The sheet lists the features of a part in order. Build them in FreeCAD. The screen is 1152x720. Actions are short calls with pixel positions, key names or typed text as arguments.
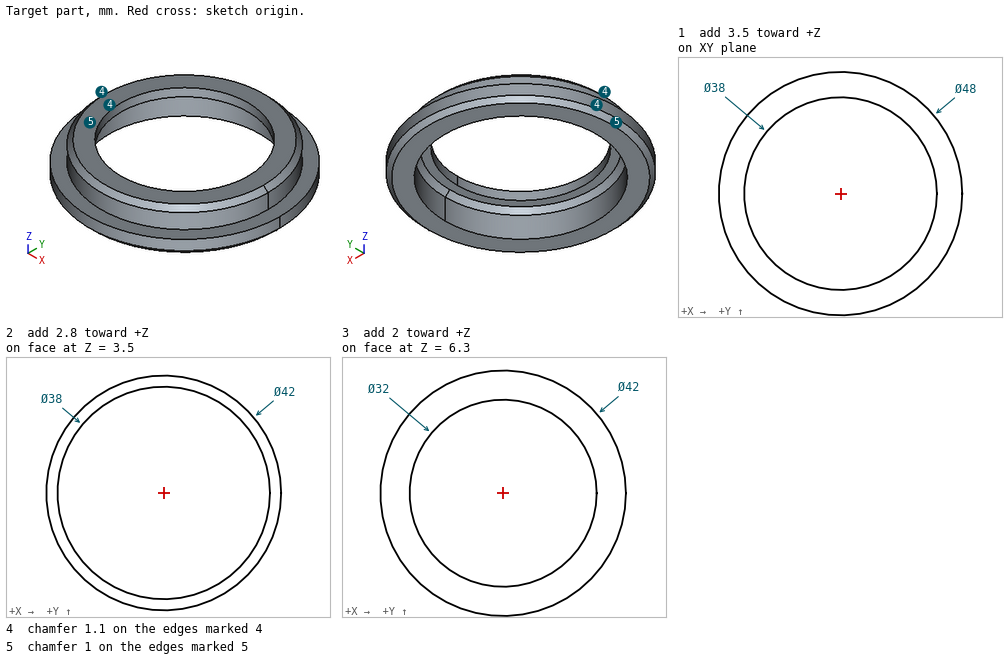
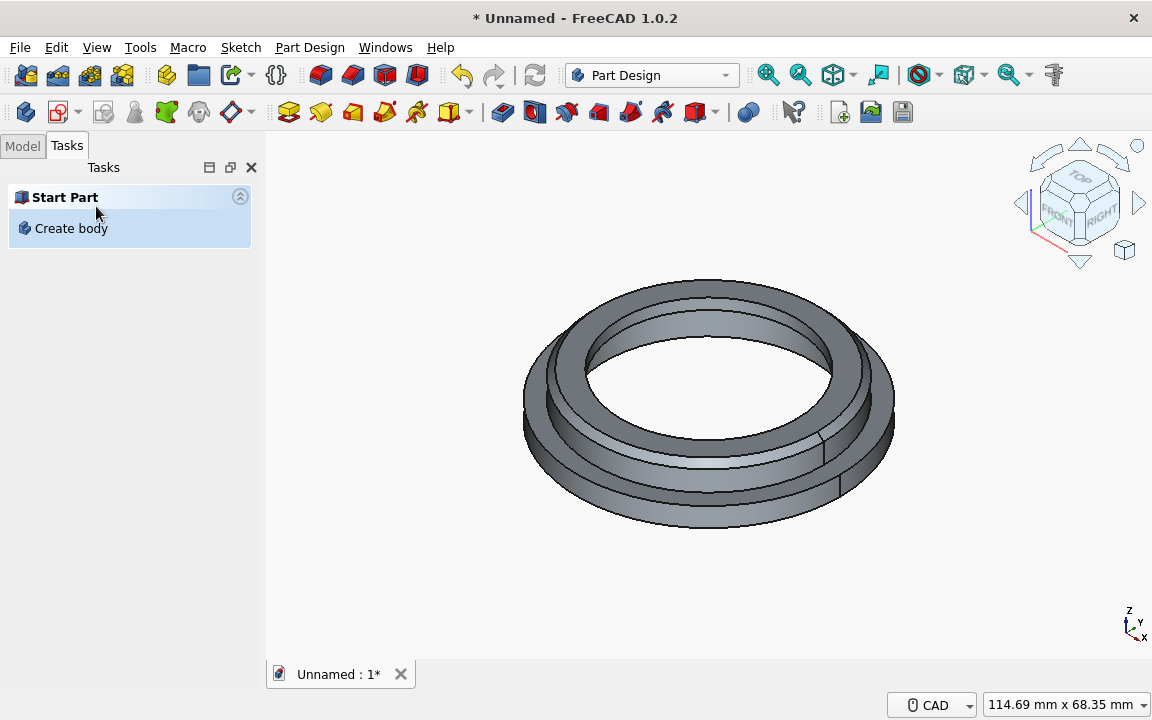
key(1)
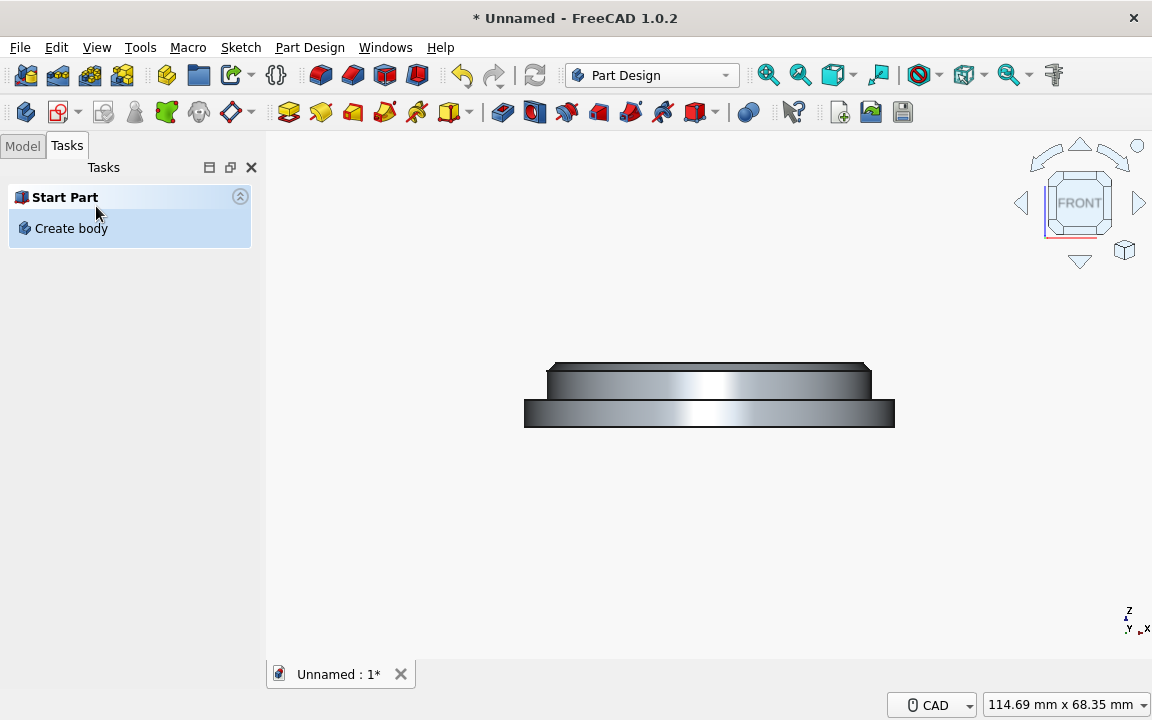
click(770, 76)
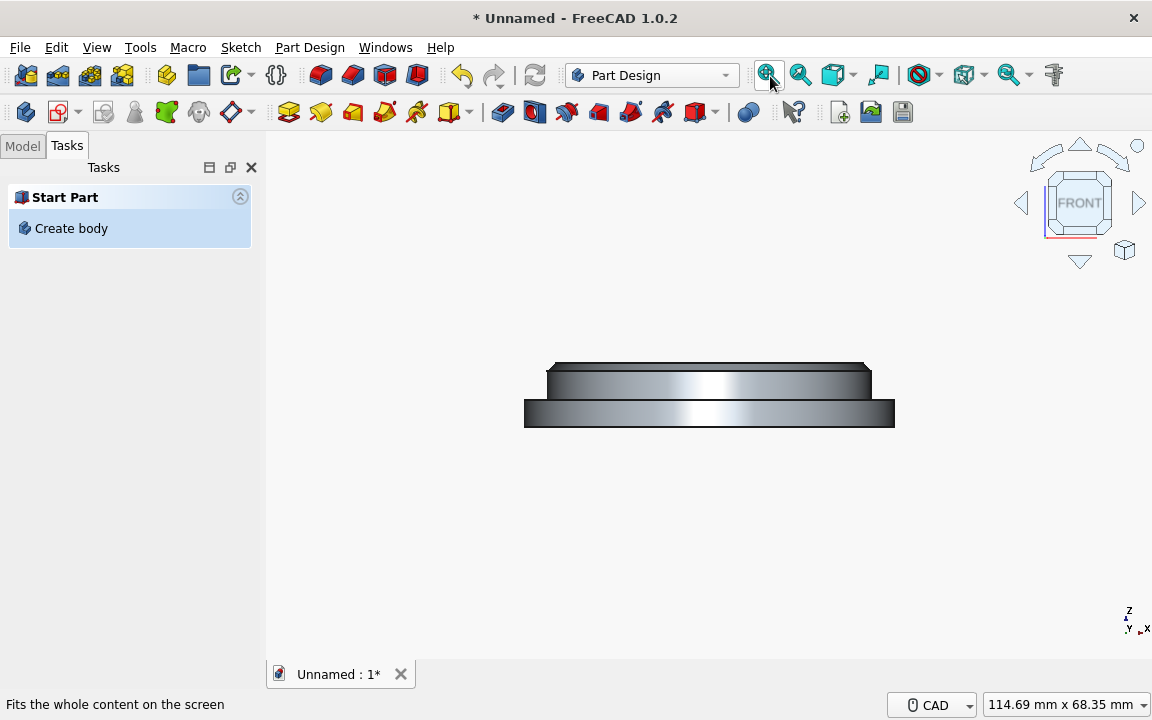
click(559, 426)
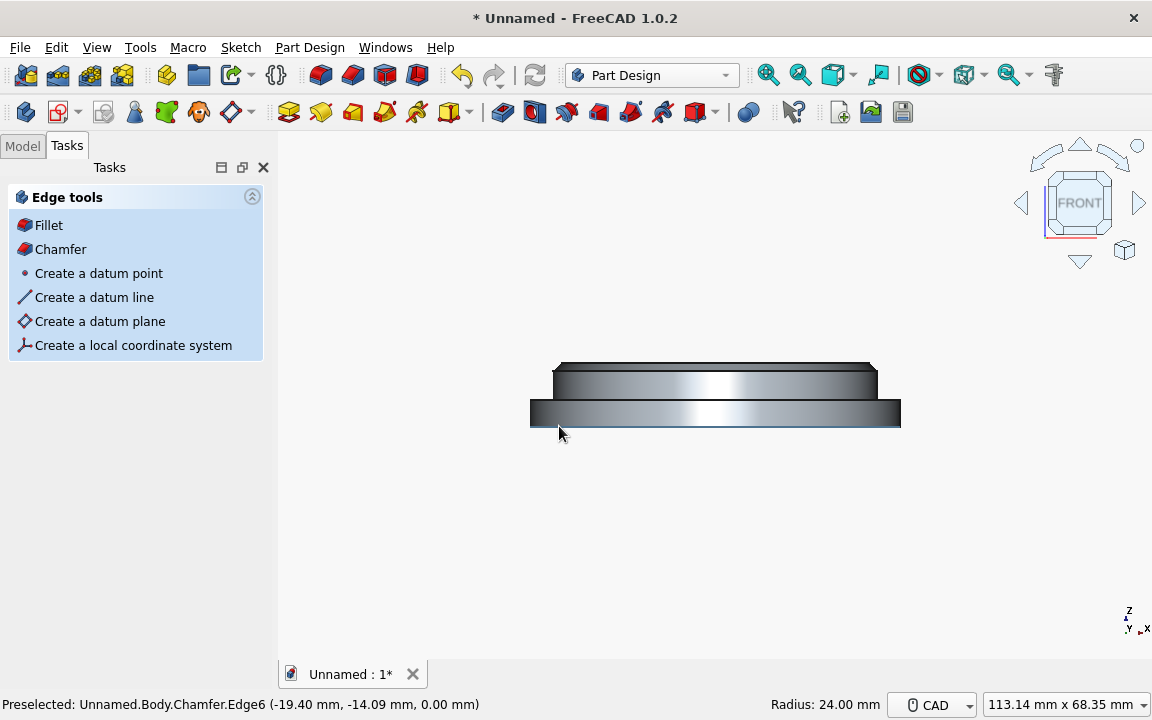
click(354, 76)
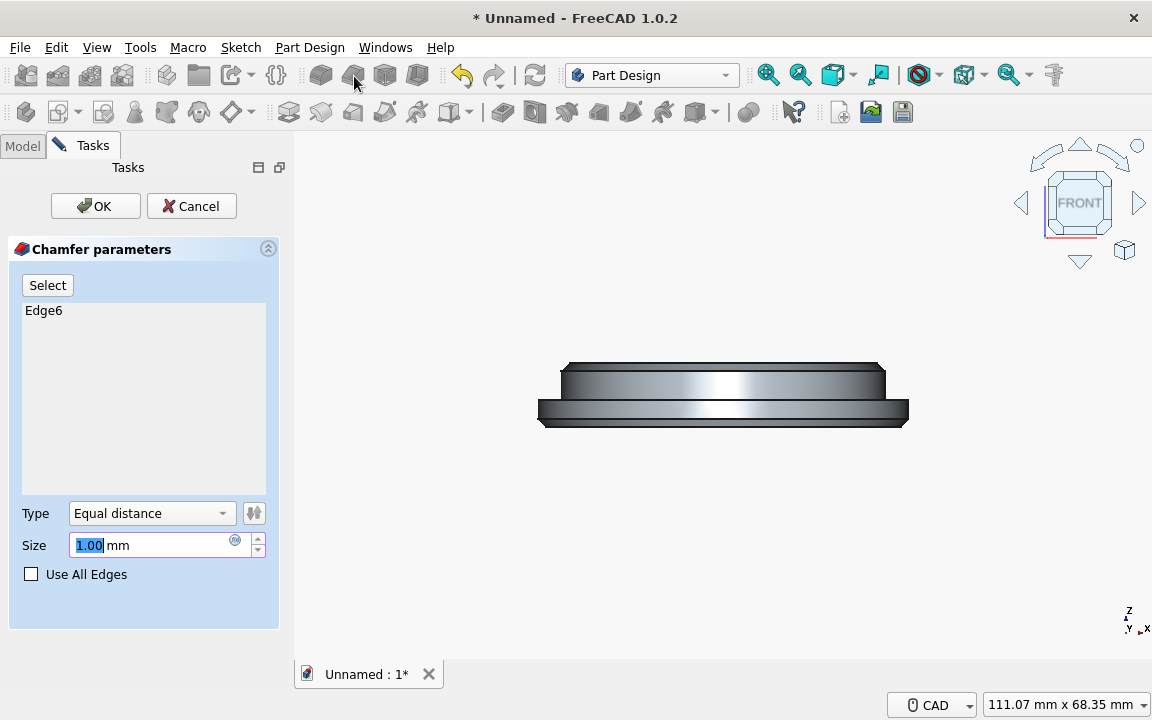
text(1)
key(Tab)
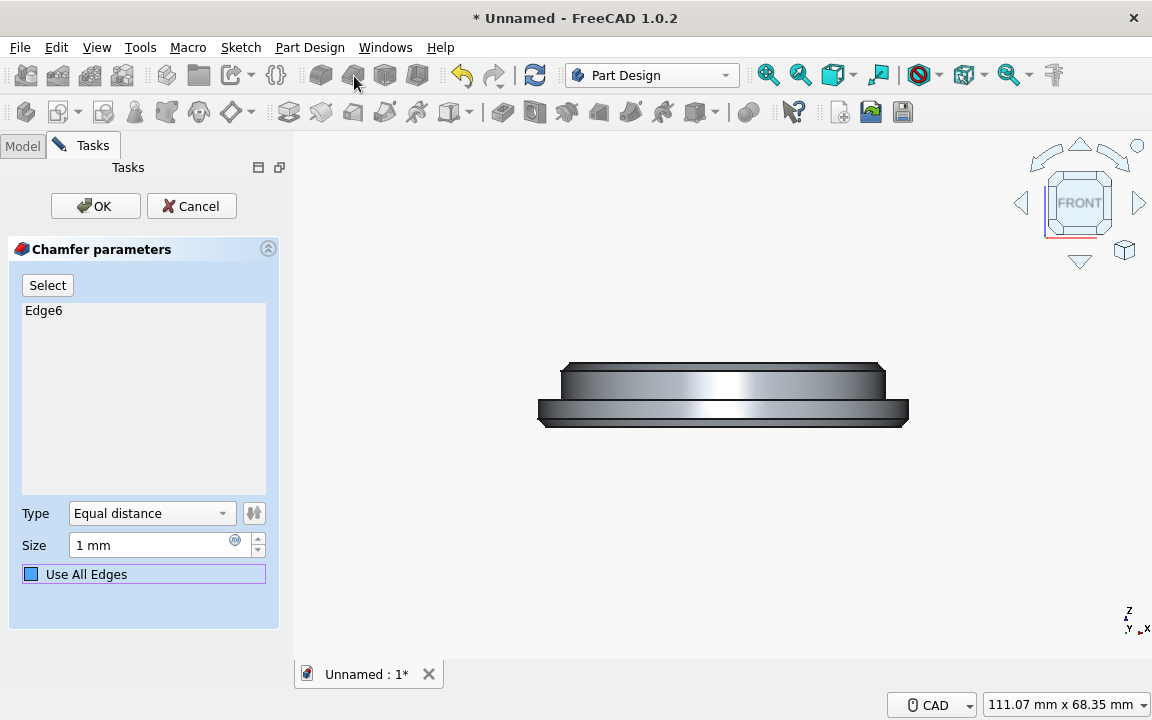
click(96, 206)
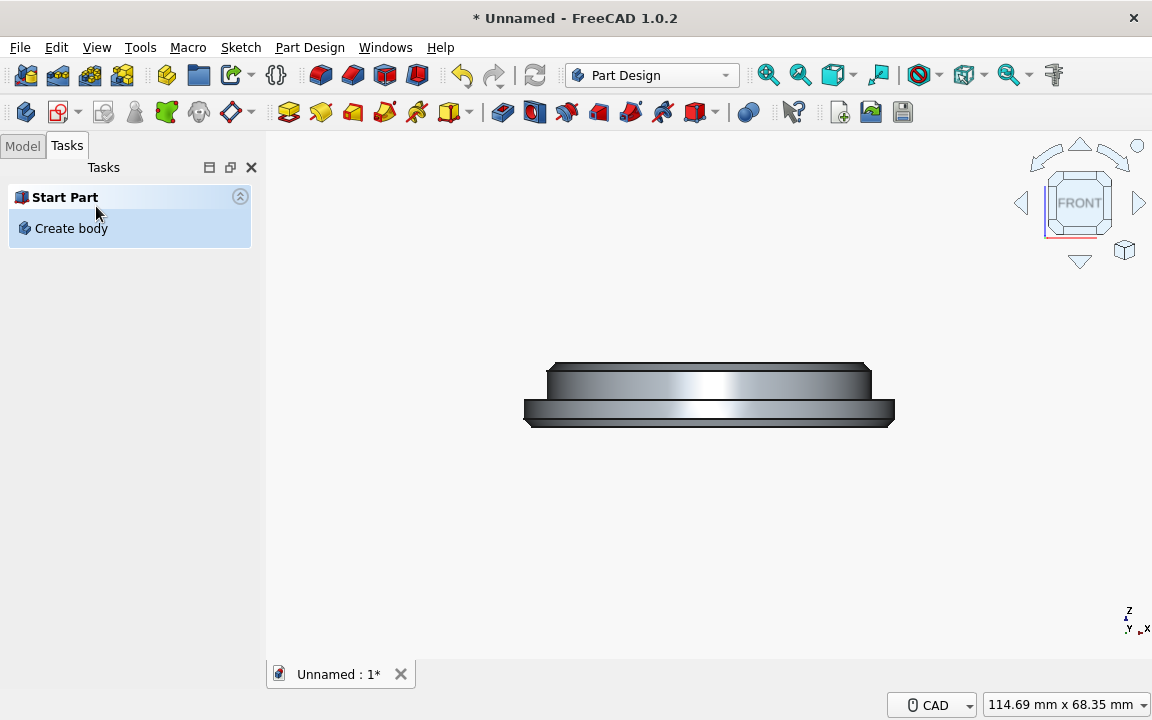
key(0)